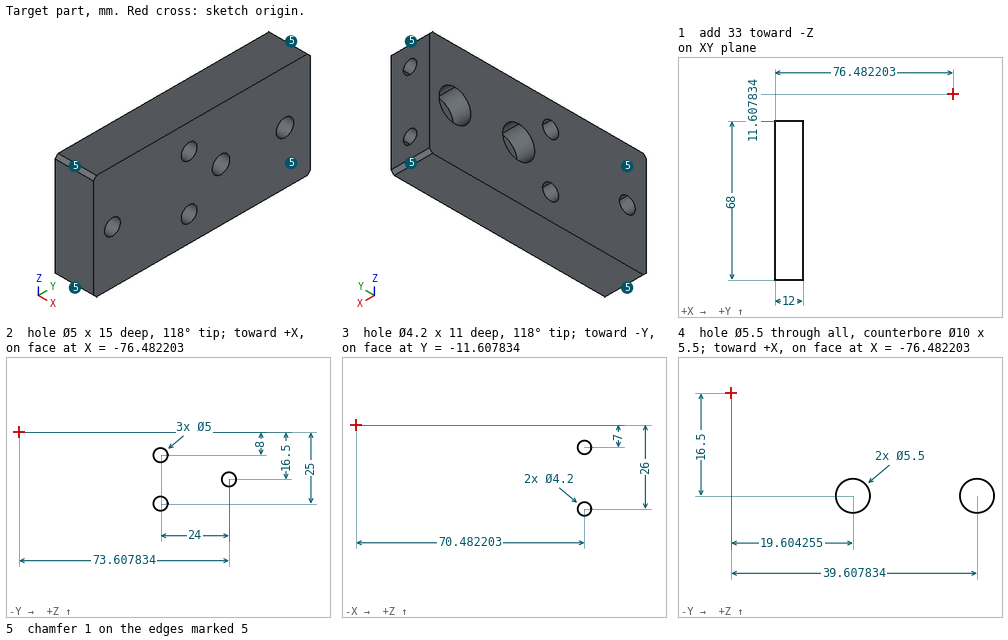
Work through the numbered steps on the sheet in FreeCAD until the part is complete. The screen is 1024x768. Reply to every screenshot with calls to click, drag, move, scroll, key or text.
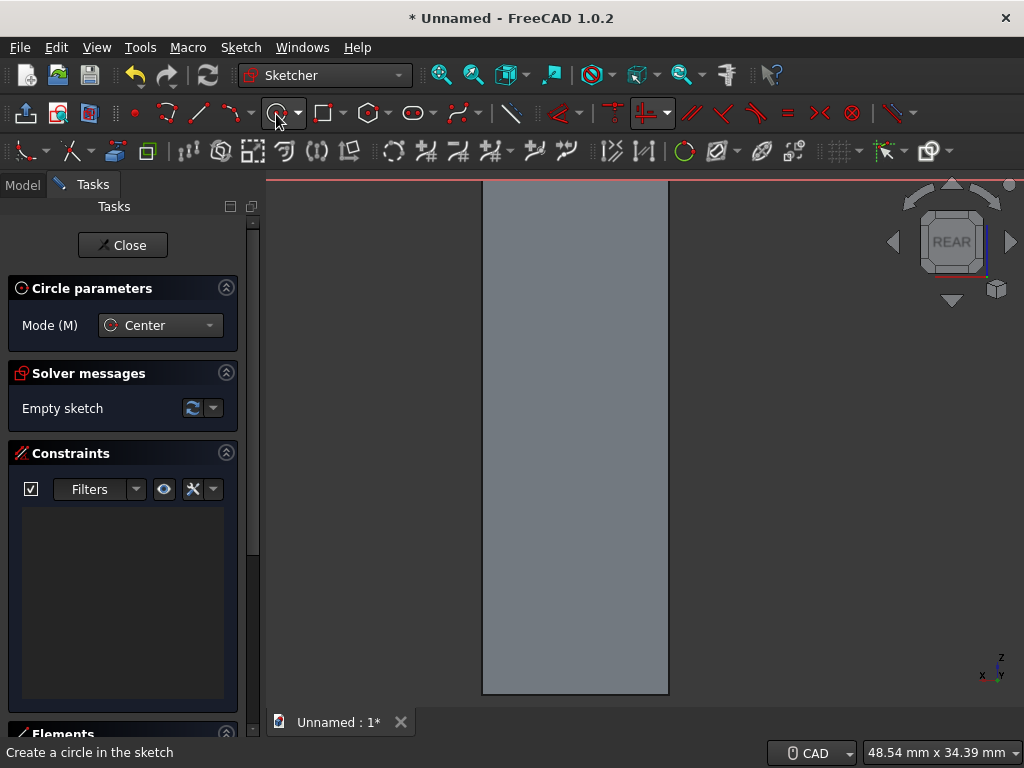
click(576, 586)
click(599, 562)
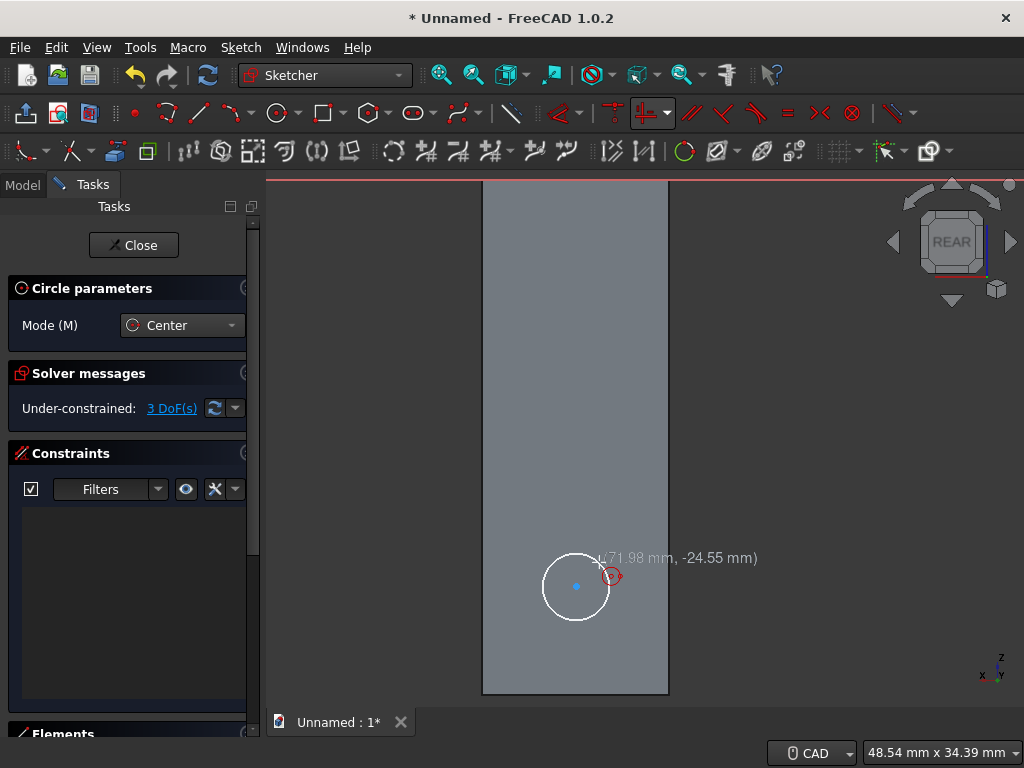
click(576, 289)
click(599, 266)
key(Escape)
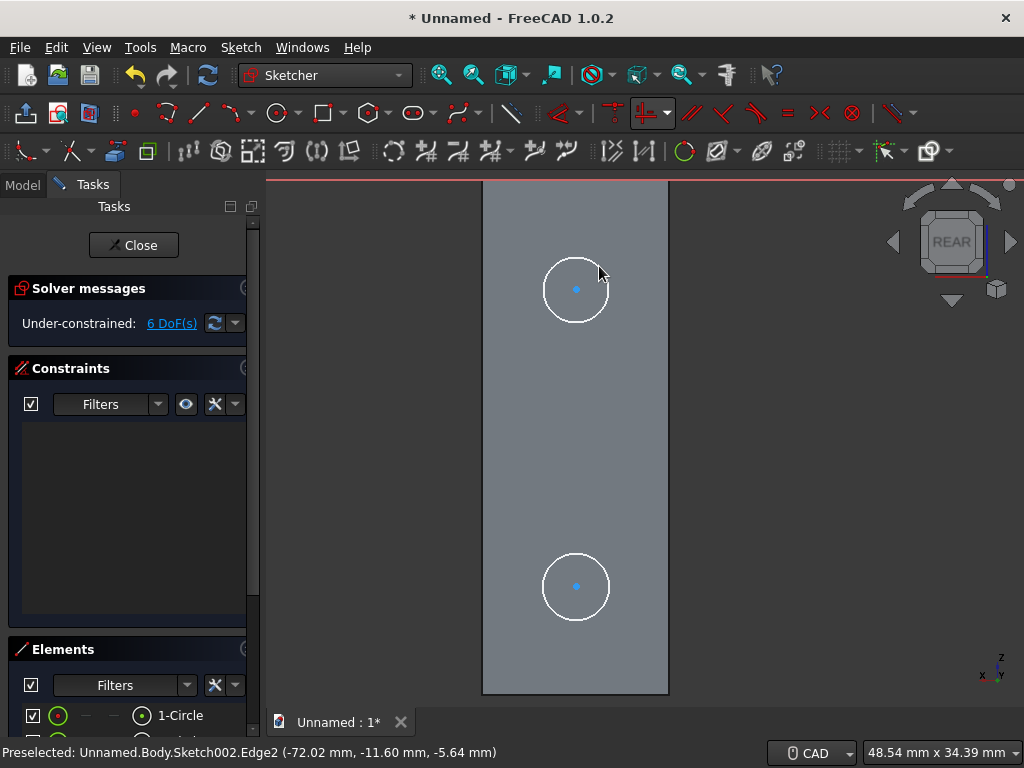
click(599, 563)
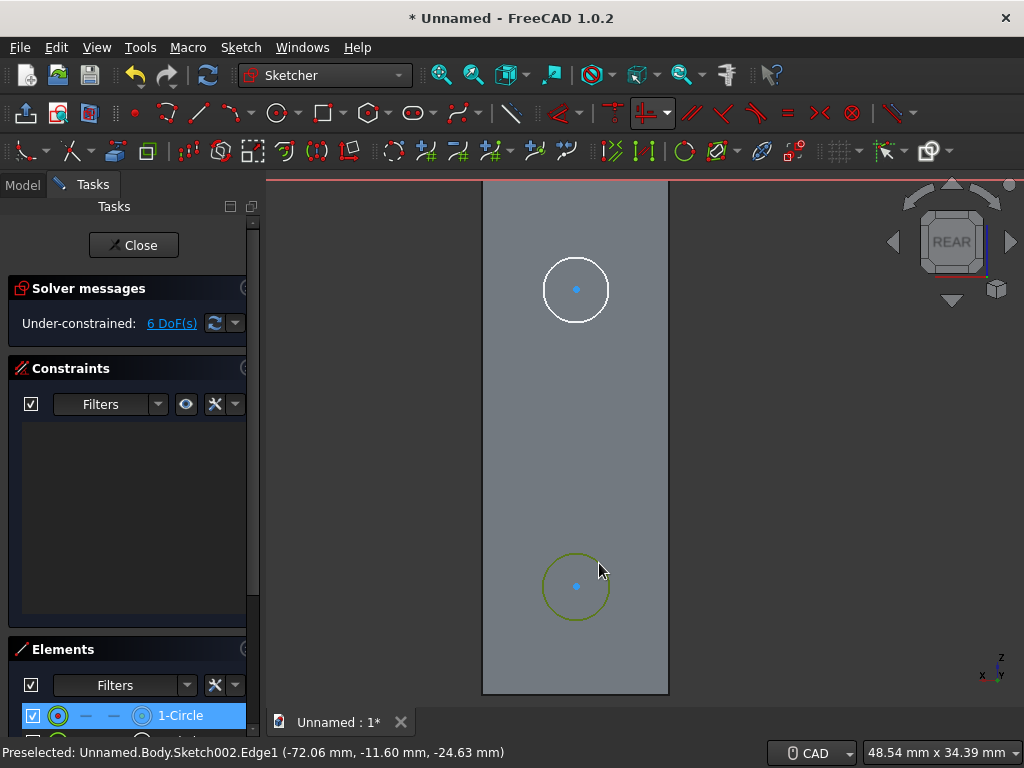
click(599, 267)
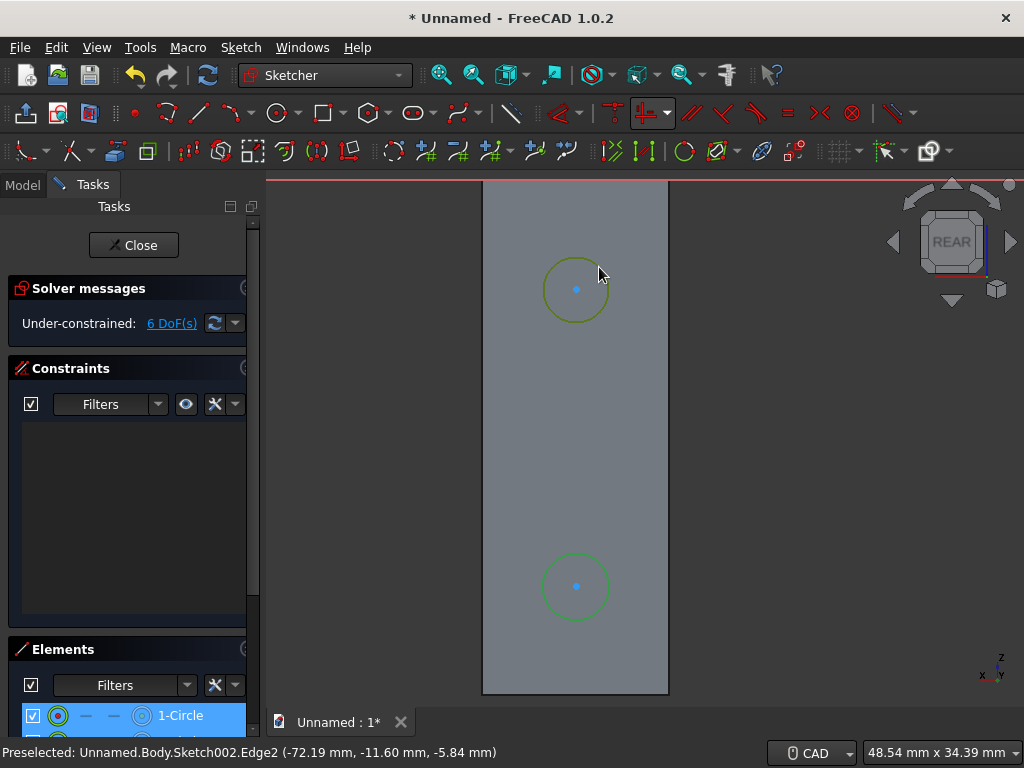
key(e)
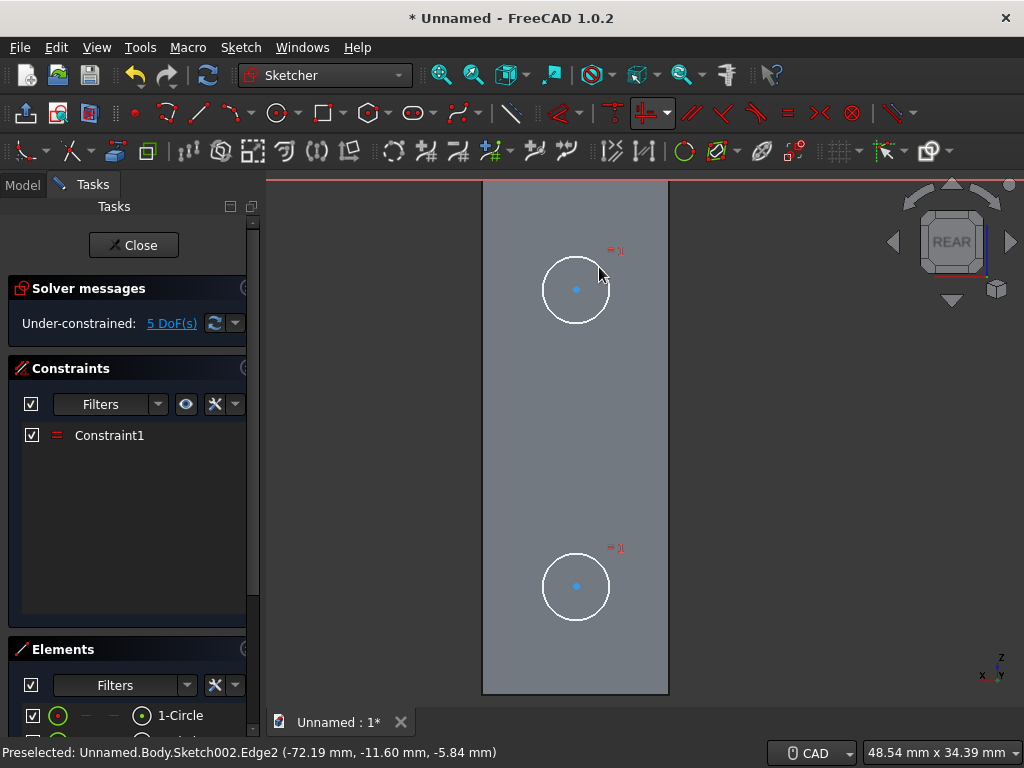
click(576, 587)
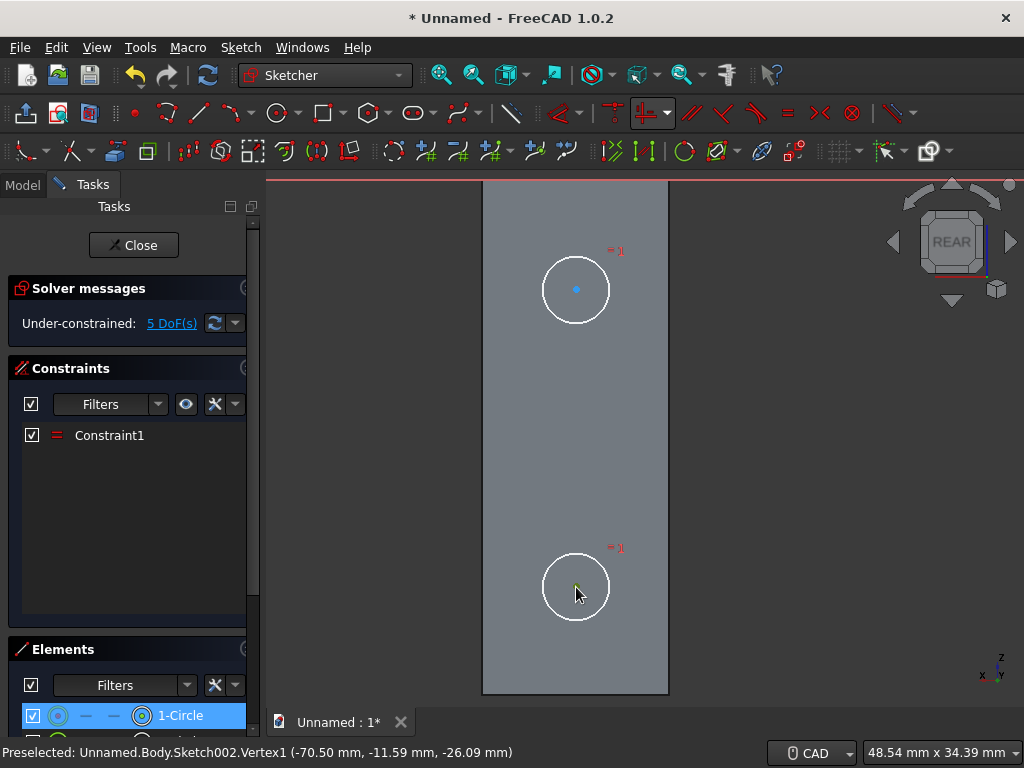
click(576, 290)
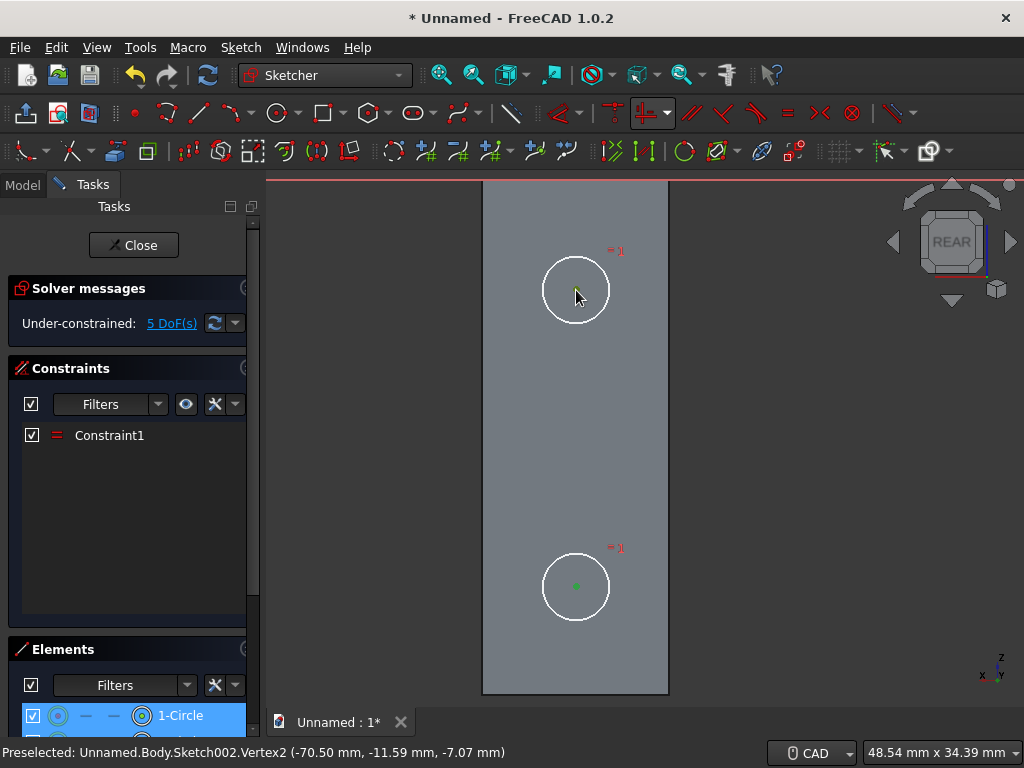
click(670, 114)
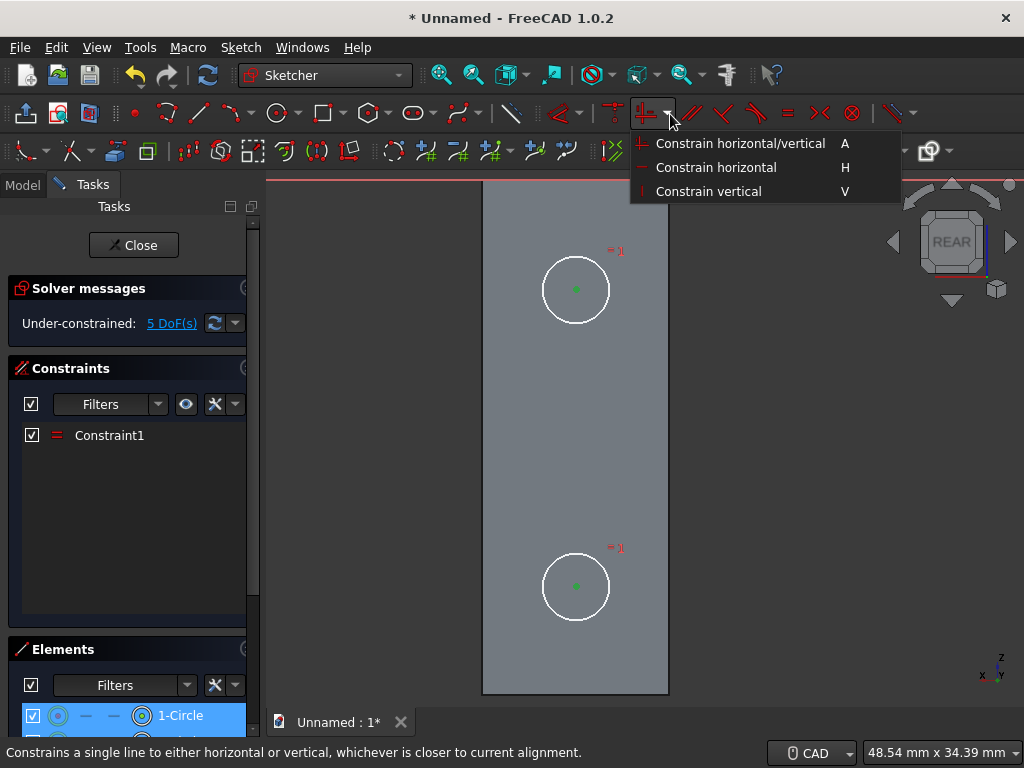
click(766, 191)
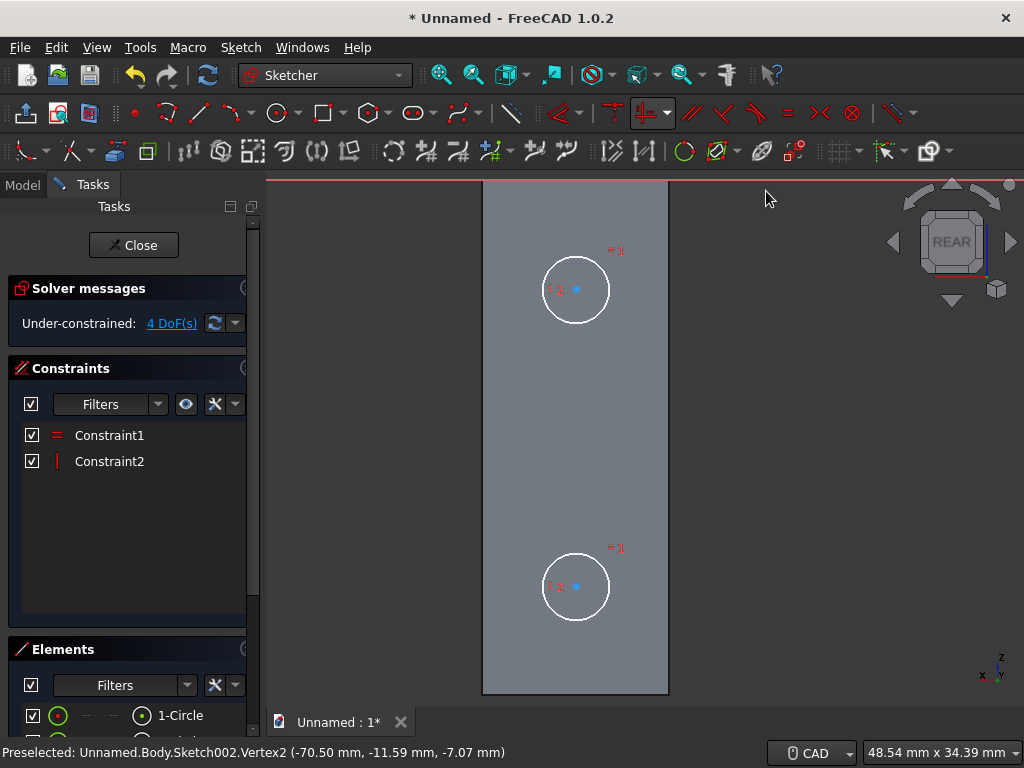
key(d)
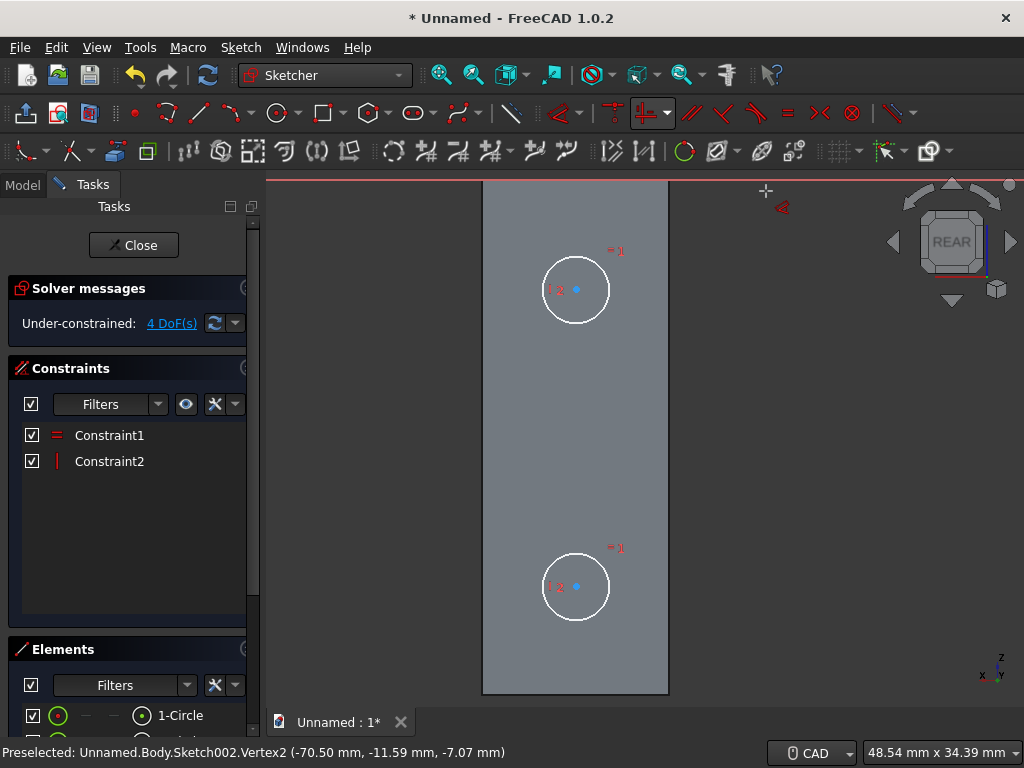
click(599, 563)
click(621, 540)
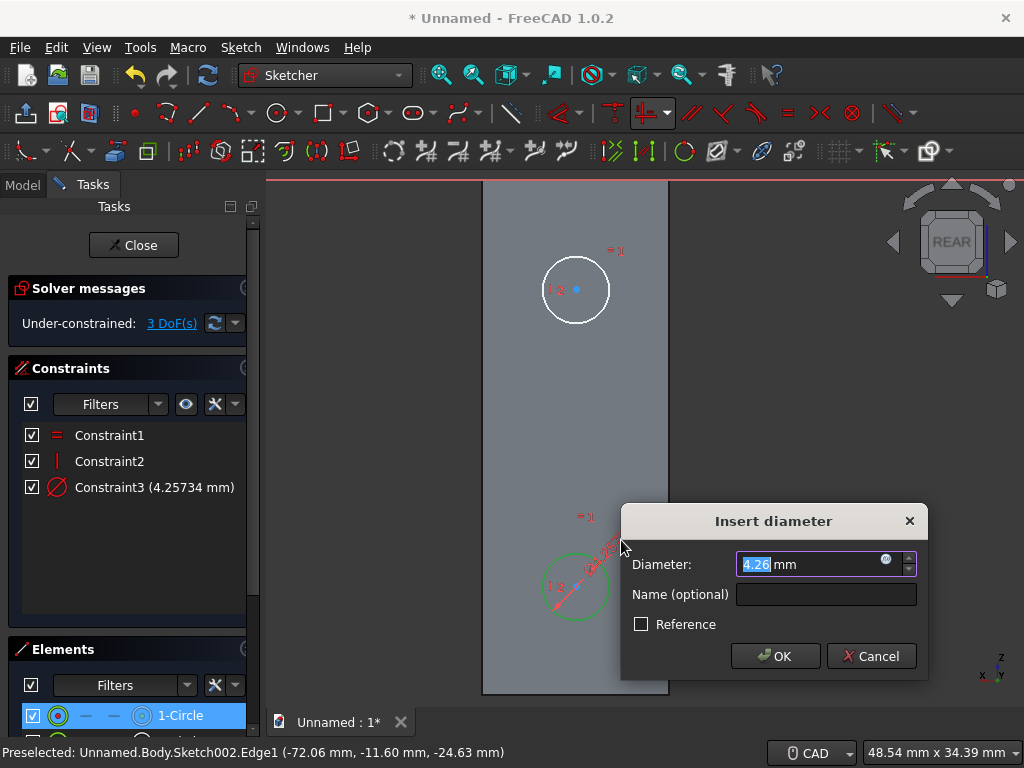
text(4.2)
key(Return)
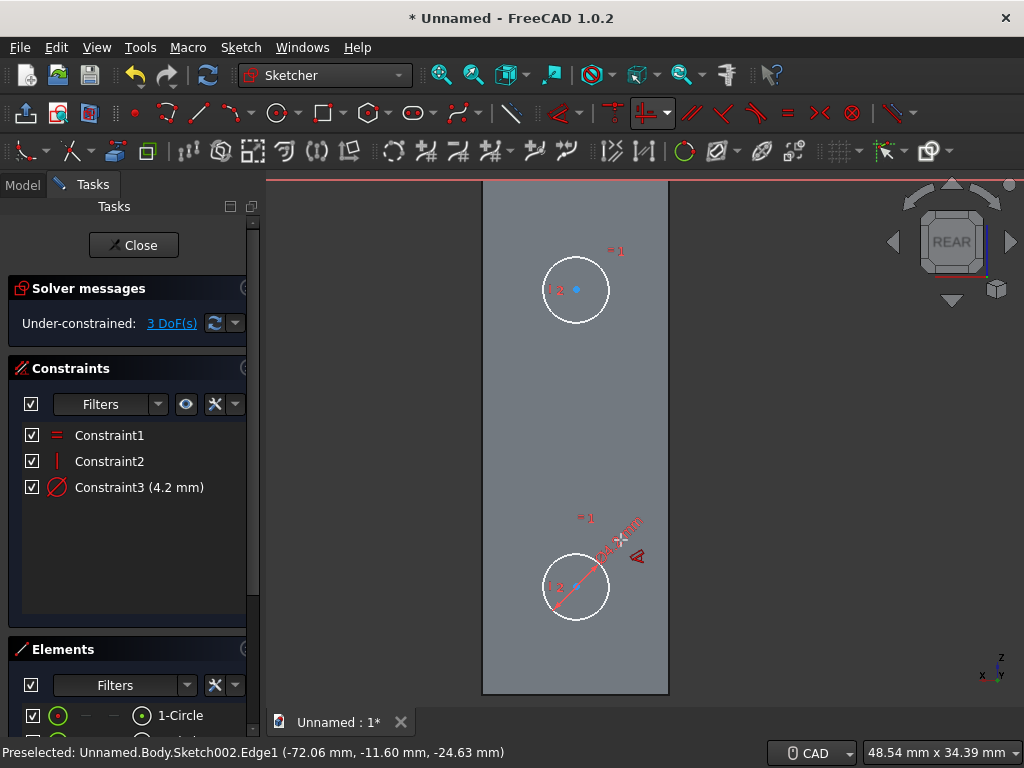
click(576, 290)
click(610, 244)